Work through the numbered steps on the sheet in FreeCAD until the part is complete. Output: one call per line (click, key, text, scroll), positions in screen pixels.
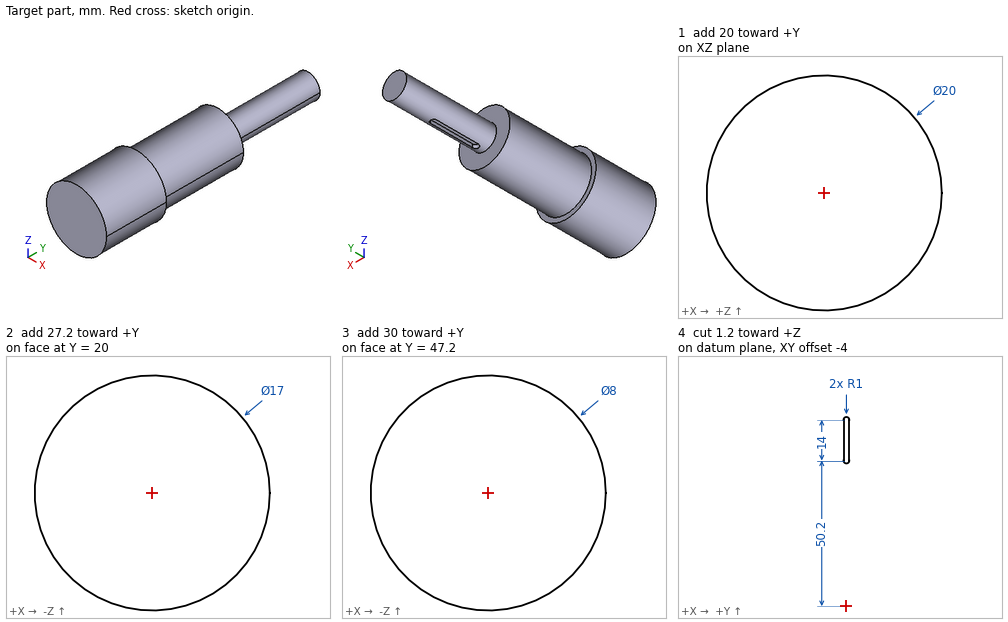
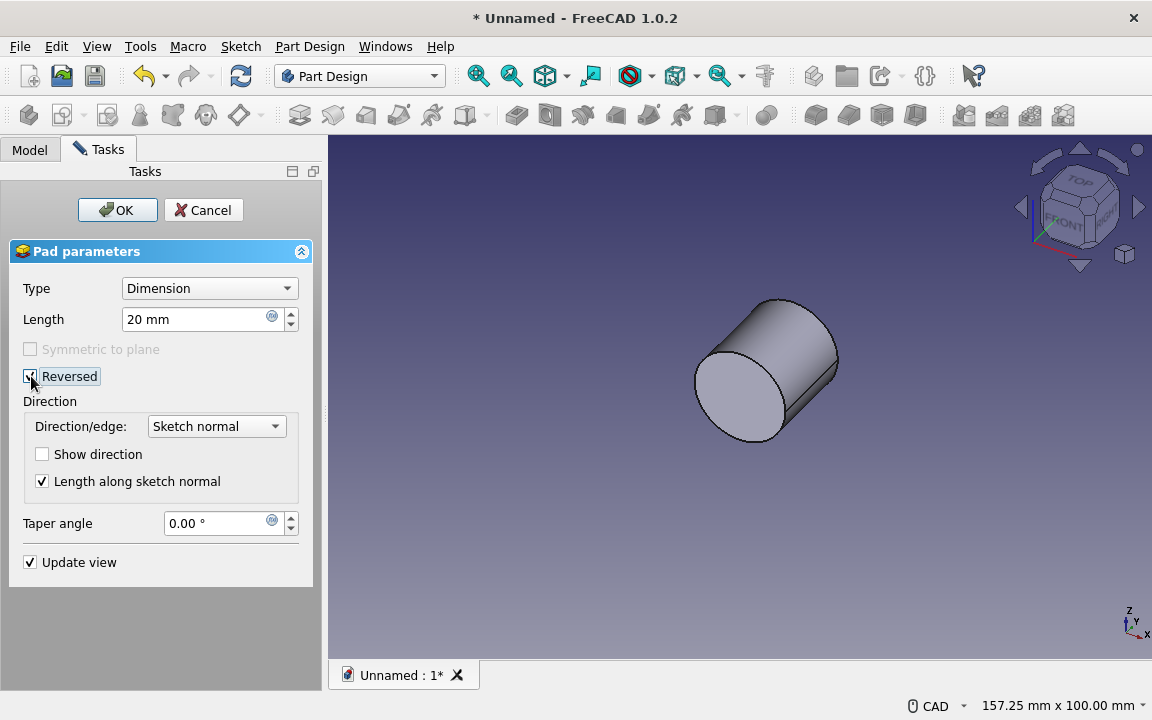
click(118, 210)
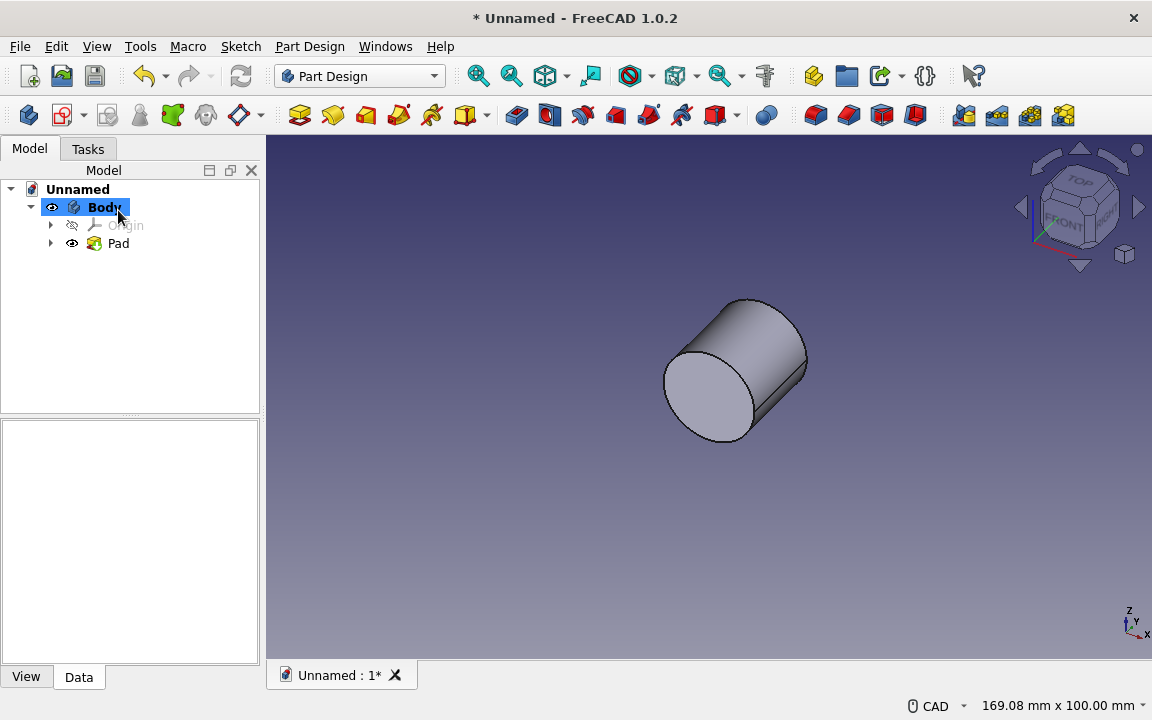
click(479, 76)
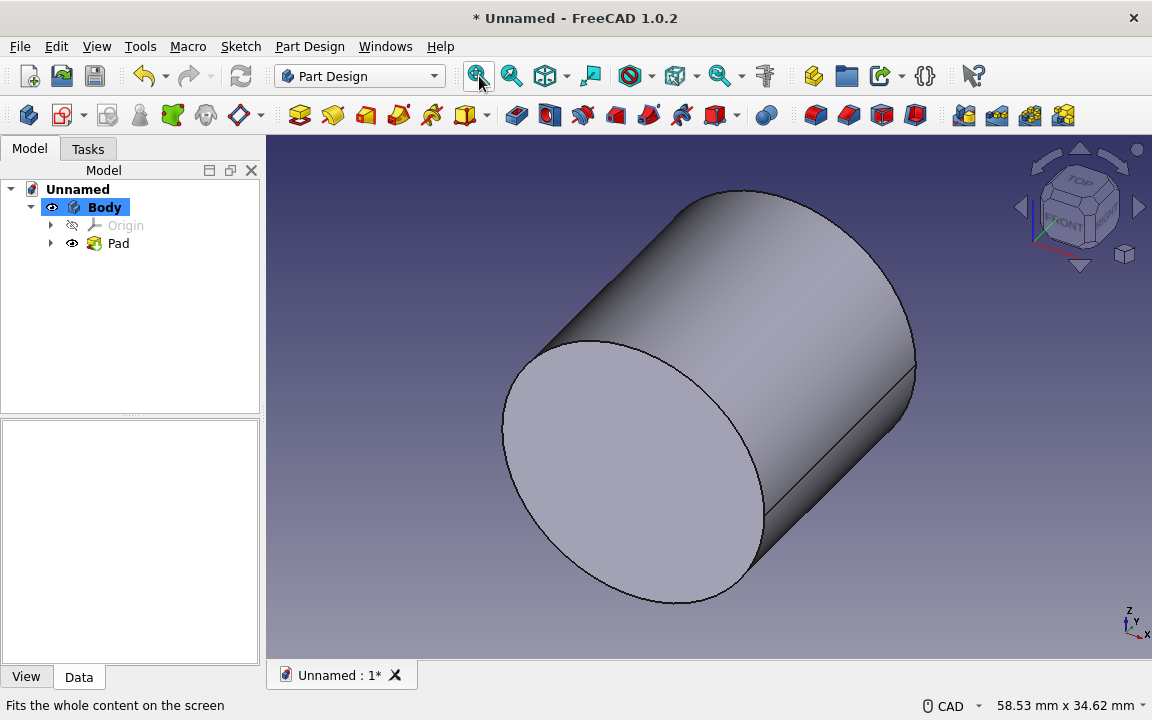
key(4)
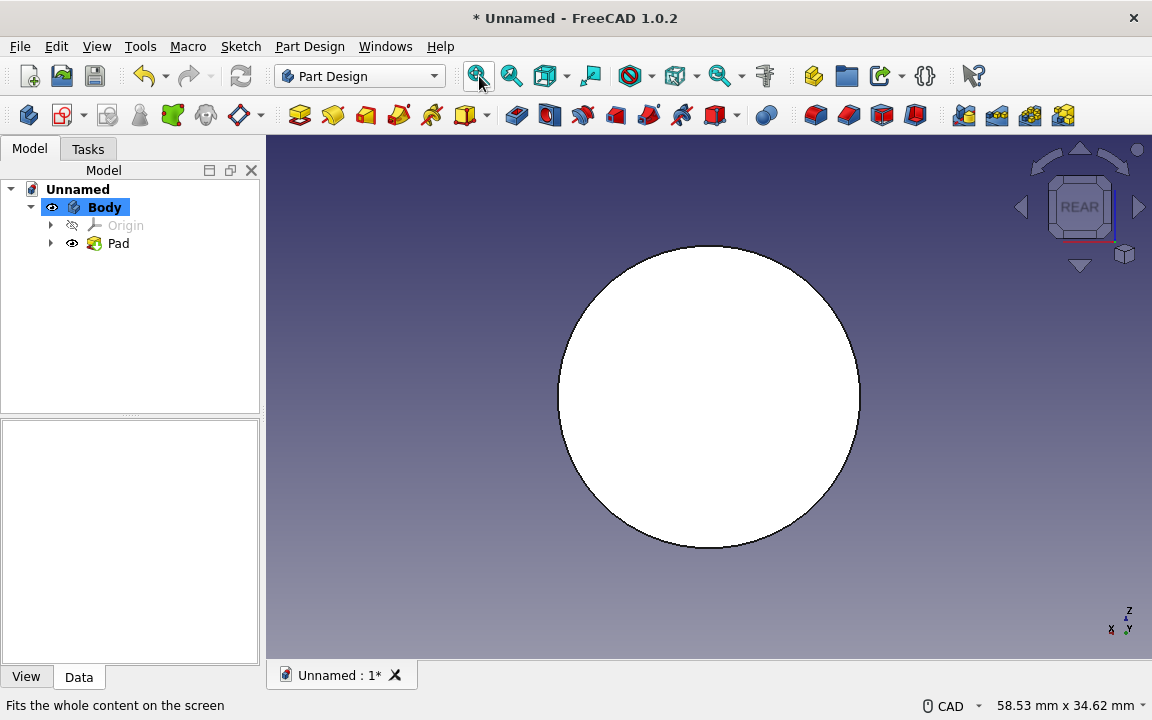
click(709, 396)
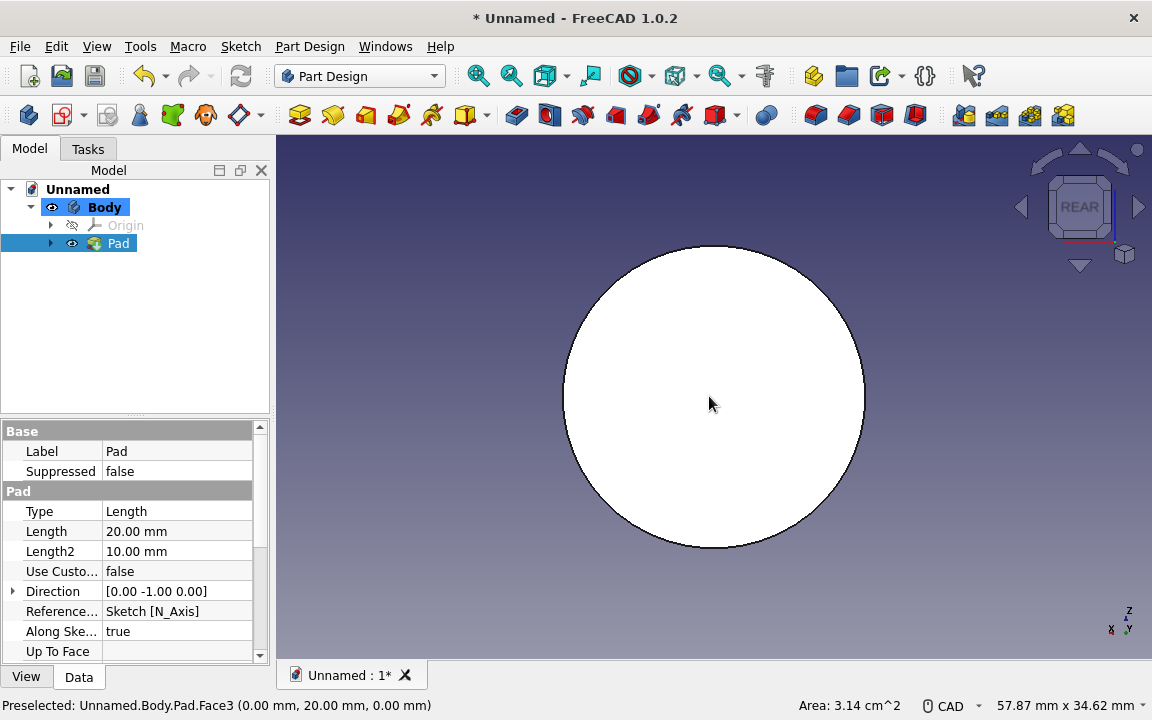
click(62, 116)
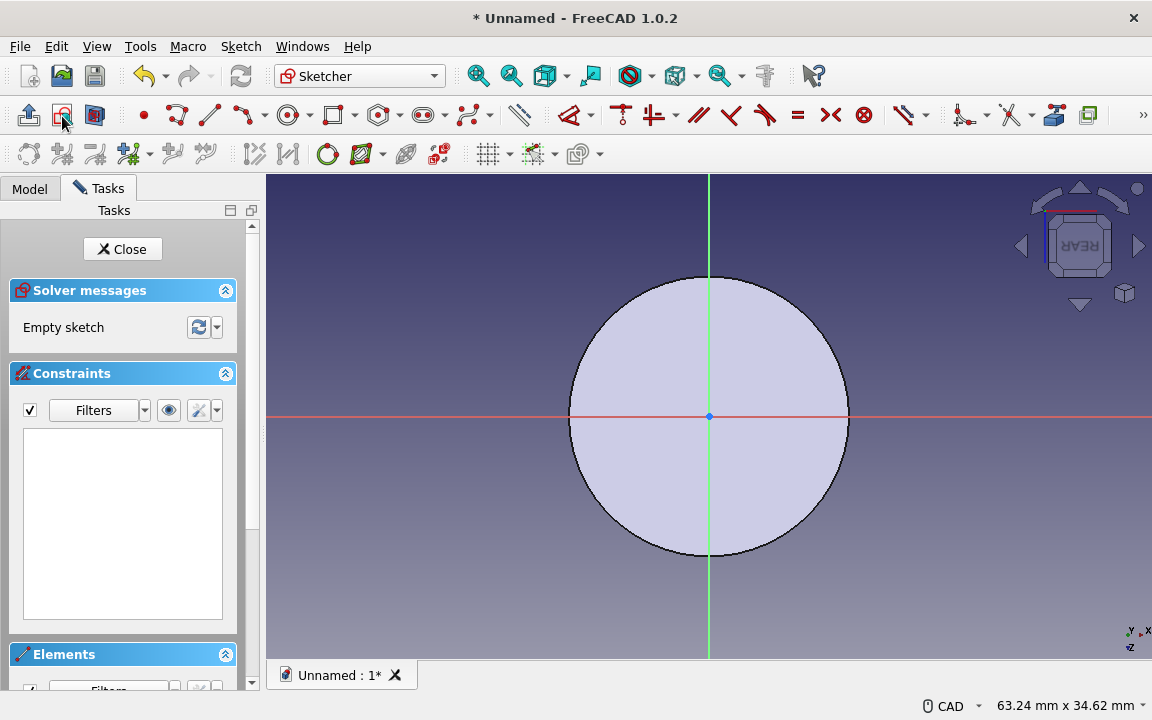
click(288, 116)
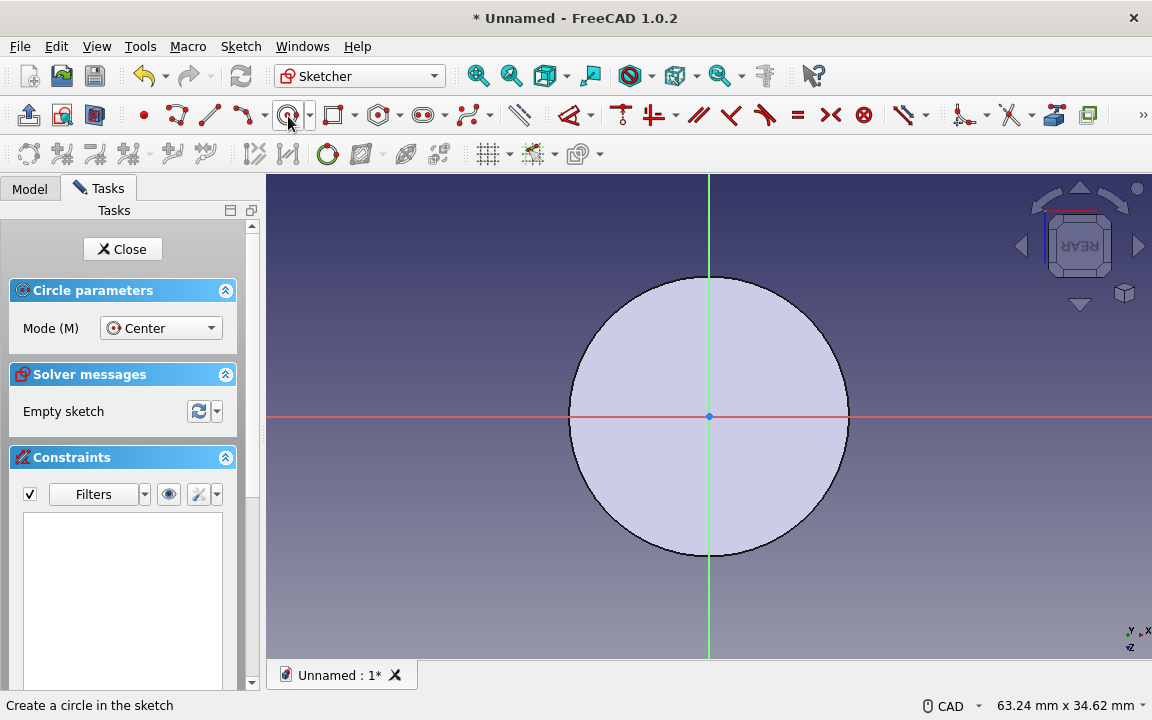
click(709, 417)
move(793, 332)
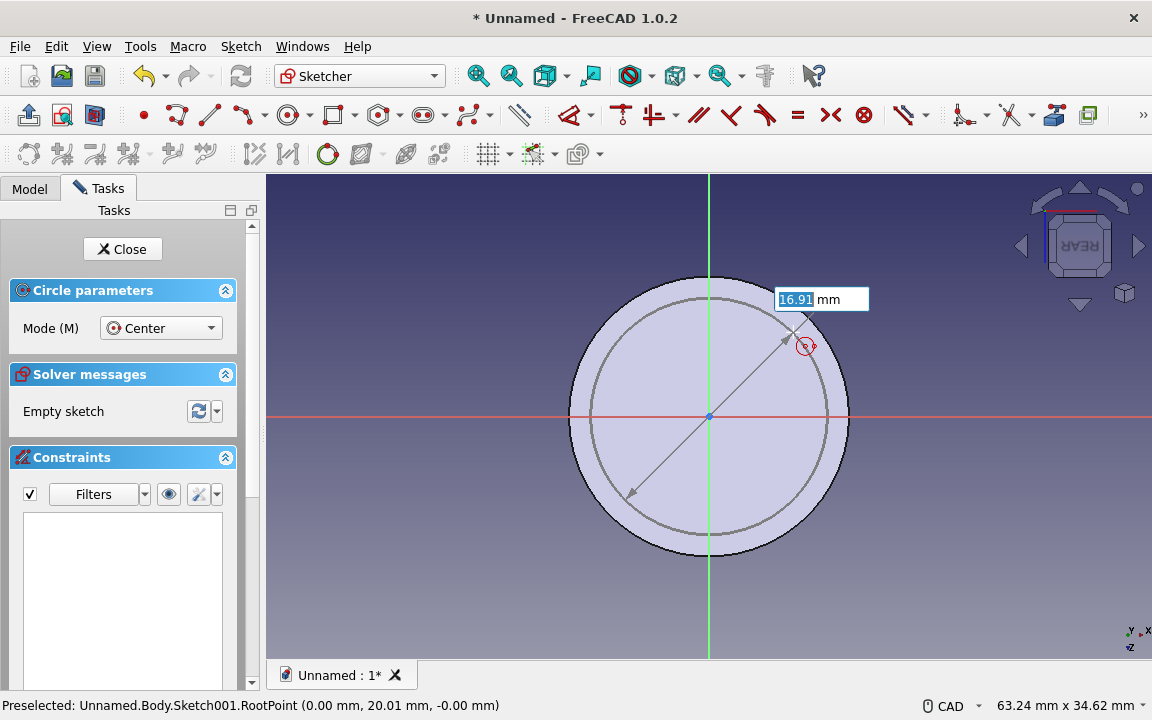
text(17)
key(Return)
key(Escape)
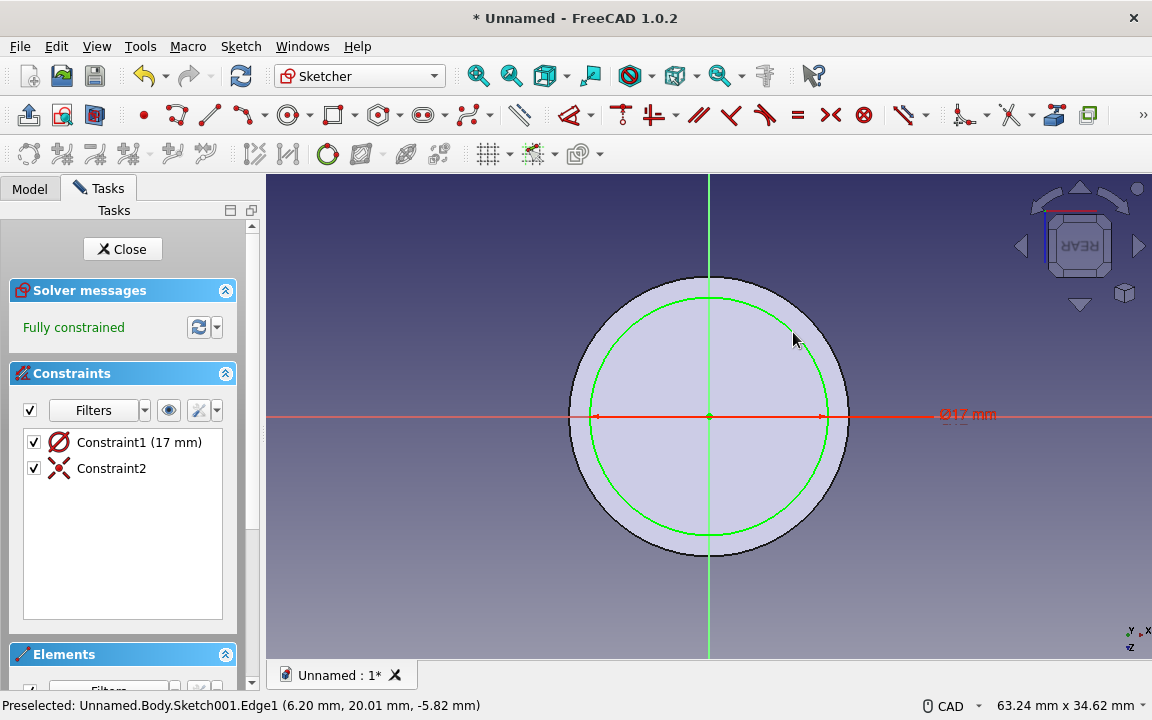
click(123, 249)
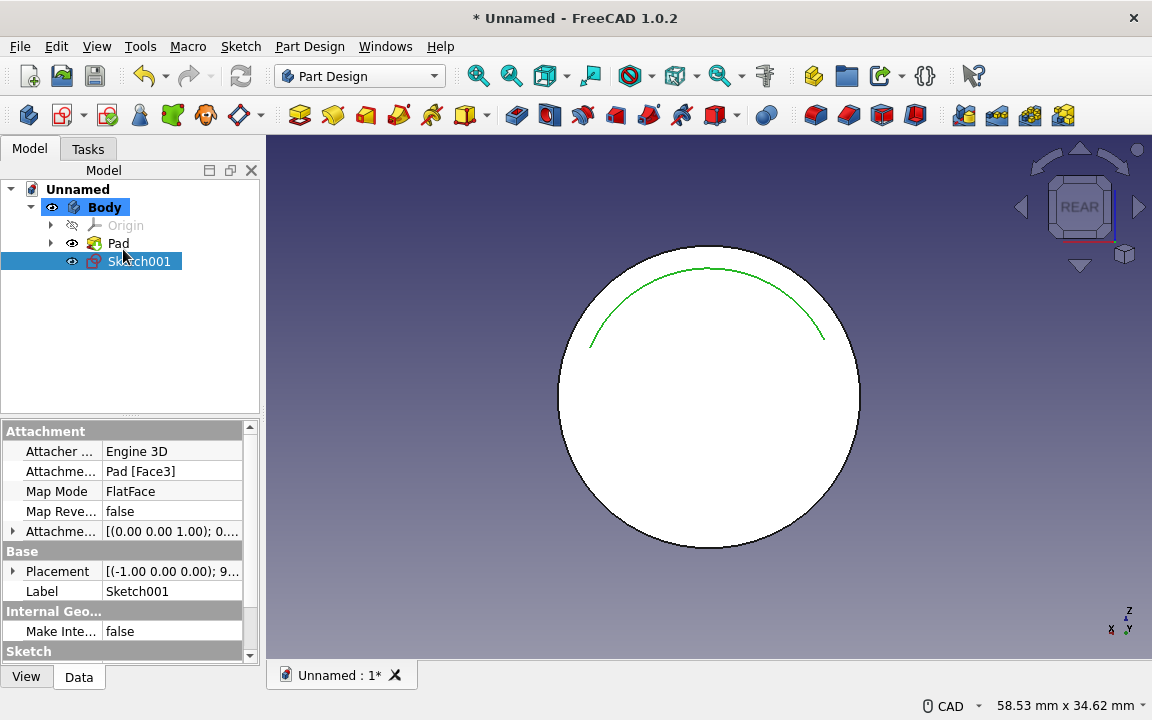
click(300, 116)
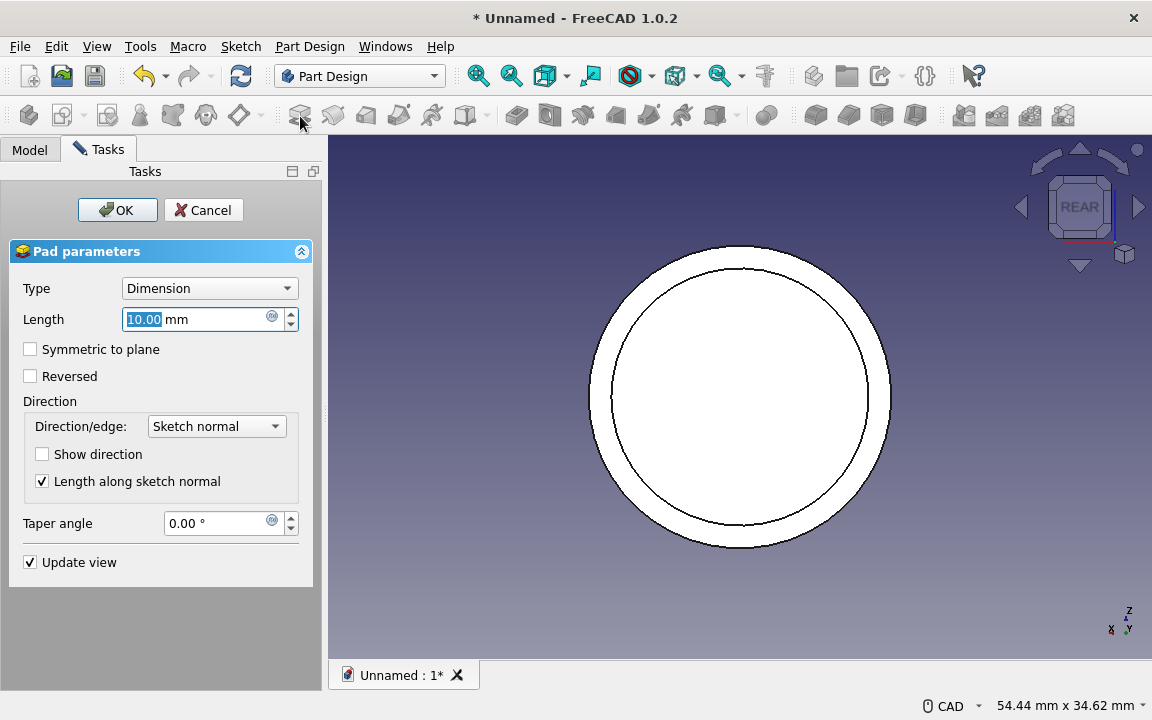
text(27.2)
key(Tab)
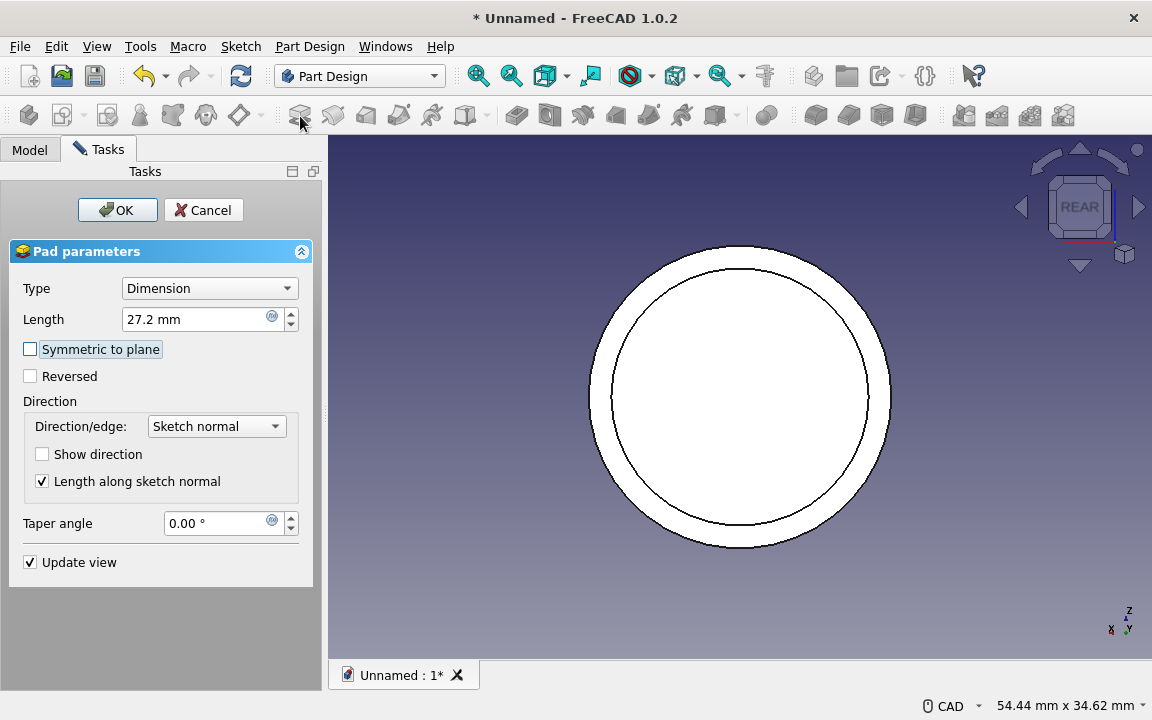
click(118, 210)